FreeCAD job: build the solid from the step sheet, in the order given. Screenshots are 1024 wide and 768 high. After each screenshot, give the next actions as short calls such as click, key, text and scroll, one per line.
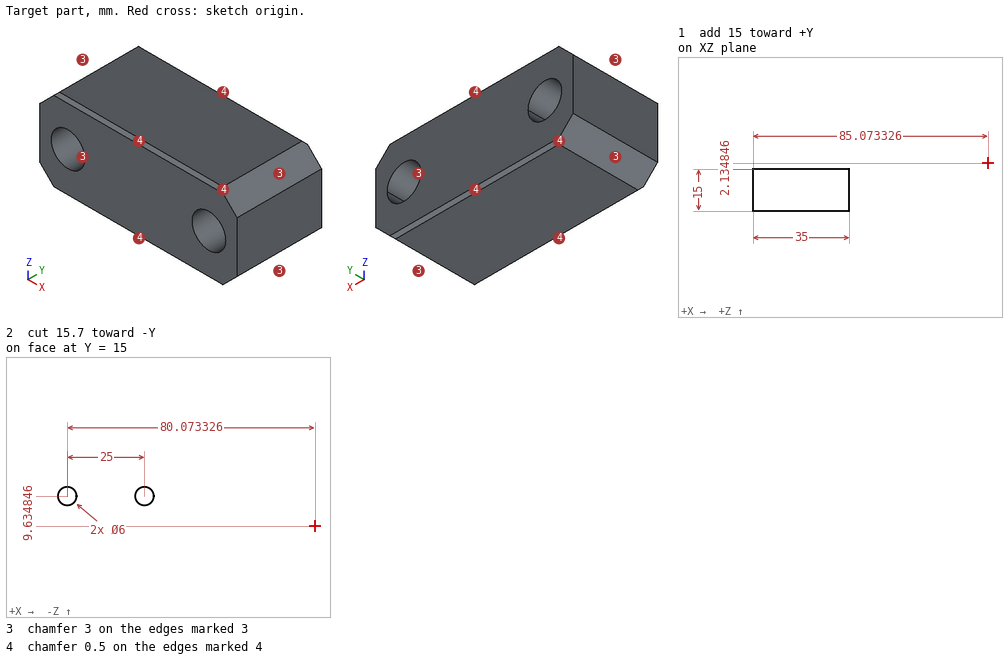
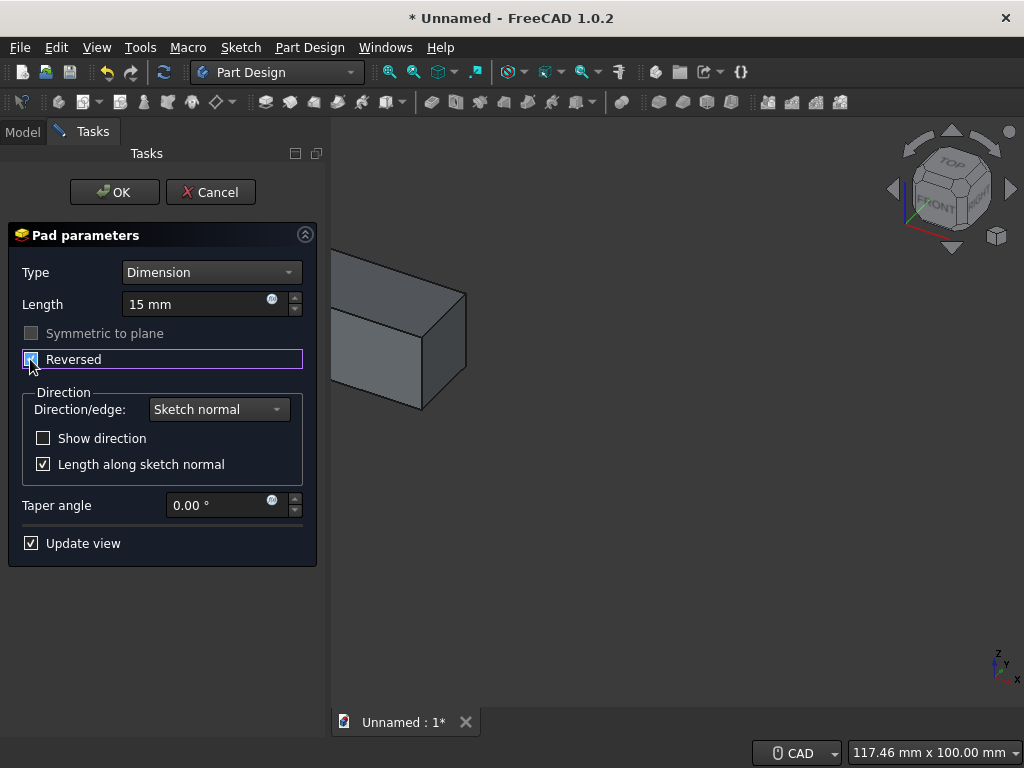
click(115, 192)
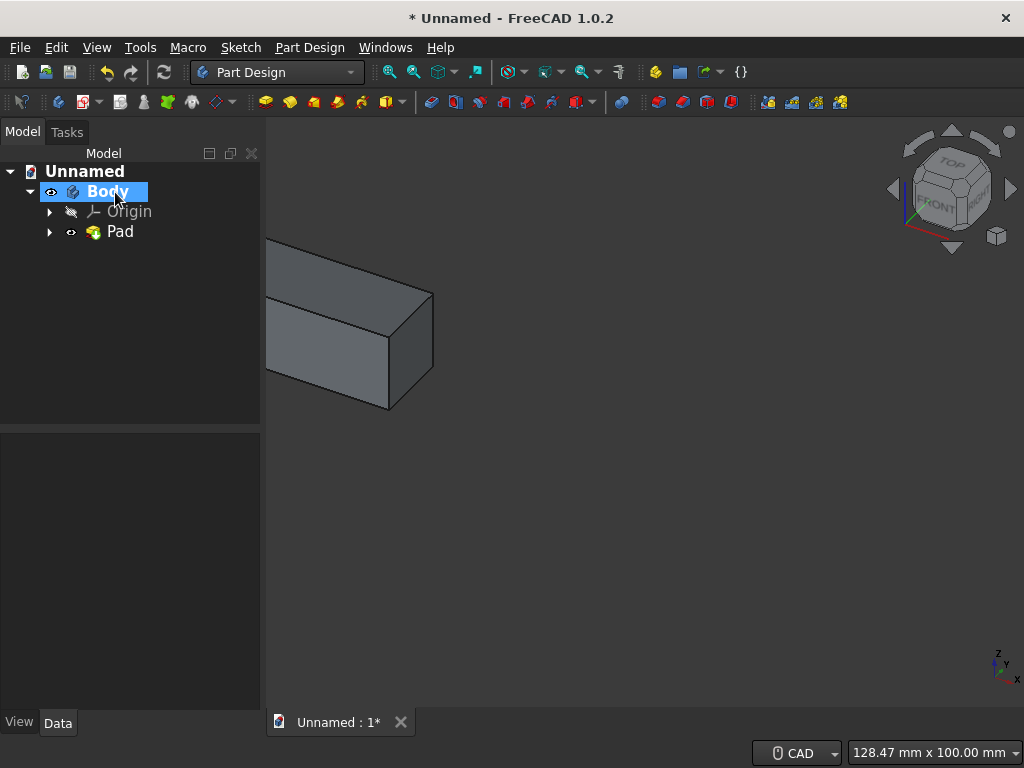
key(v)
key(f)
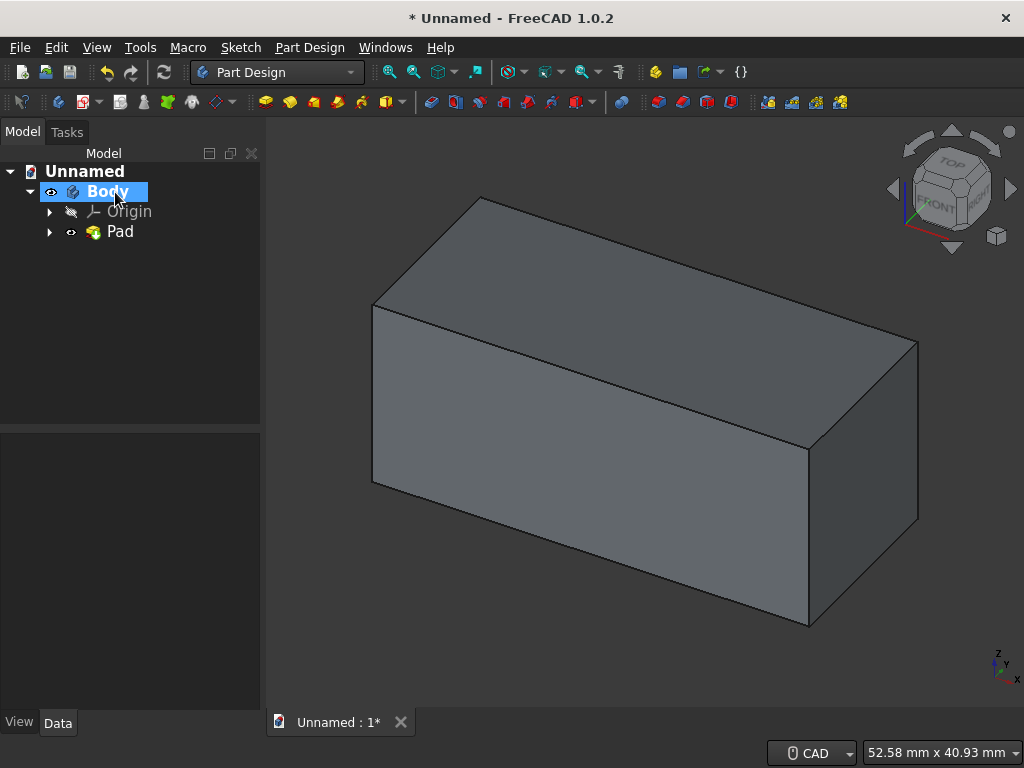
key(4)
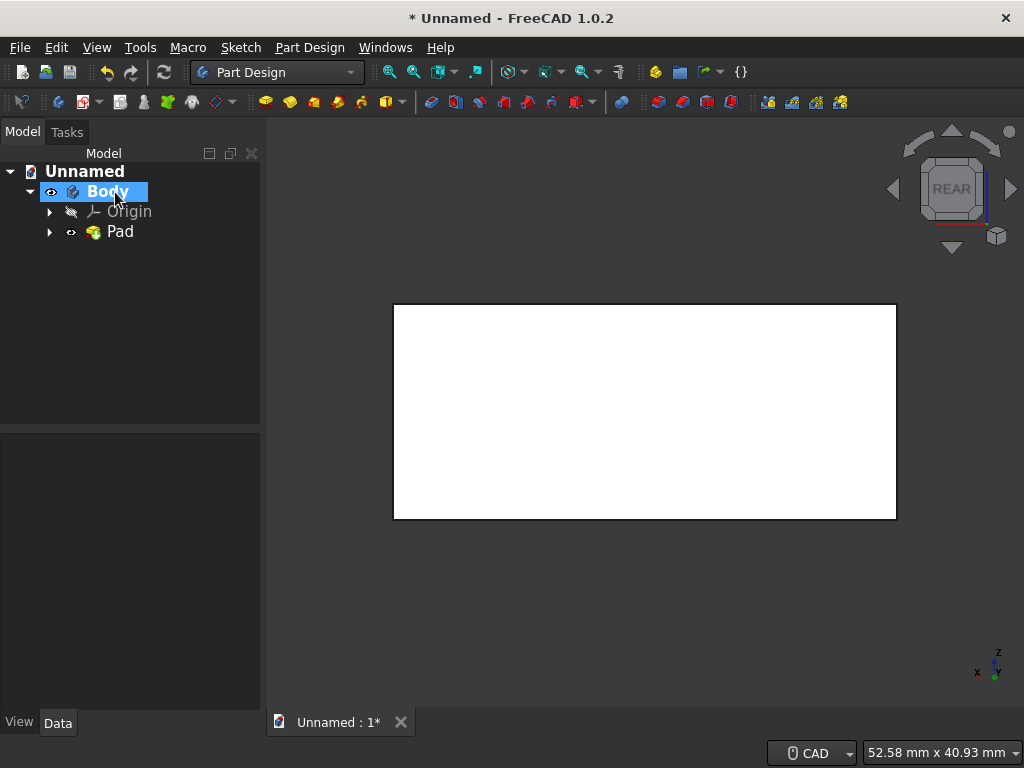
click(573, 411)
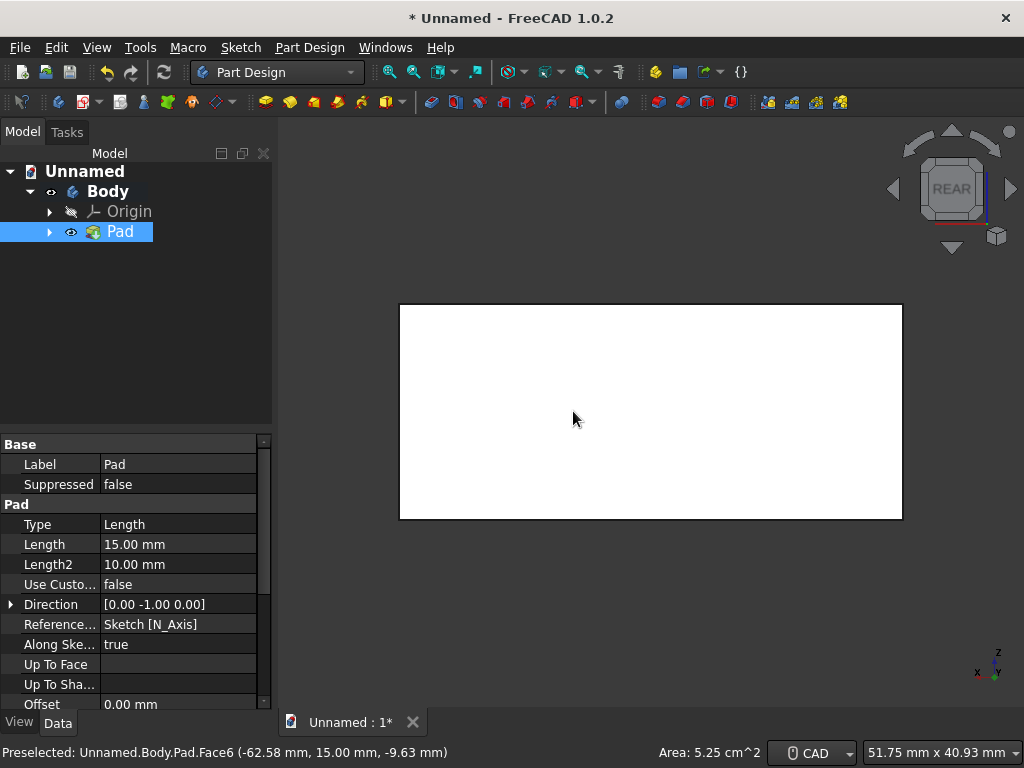
click(84, 102)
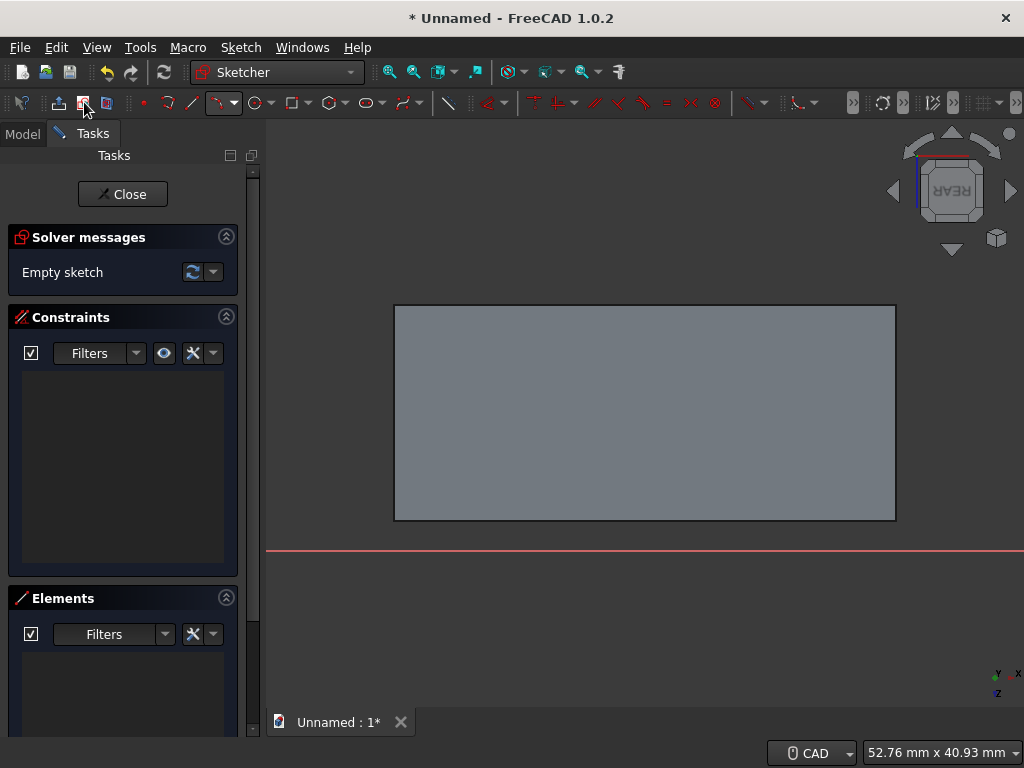
scroll(294, 413, down, 1)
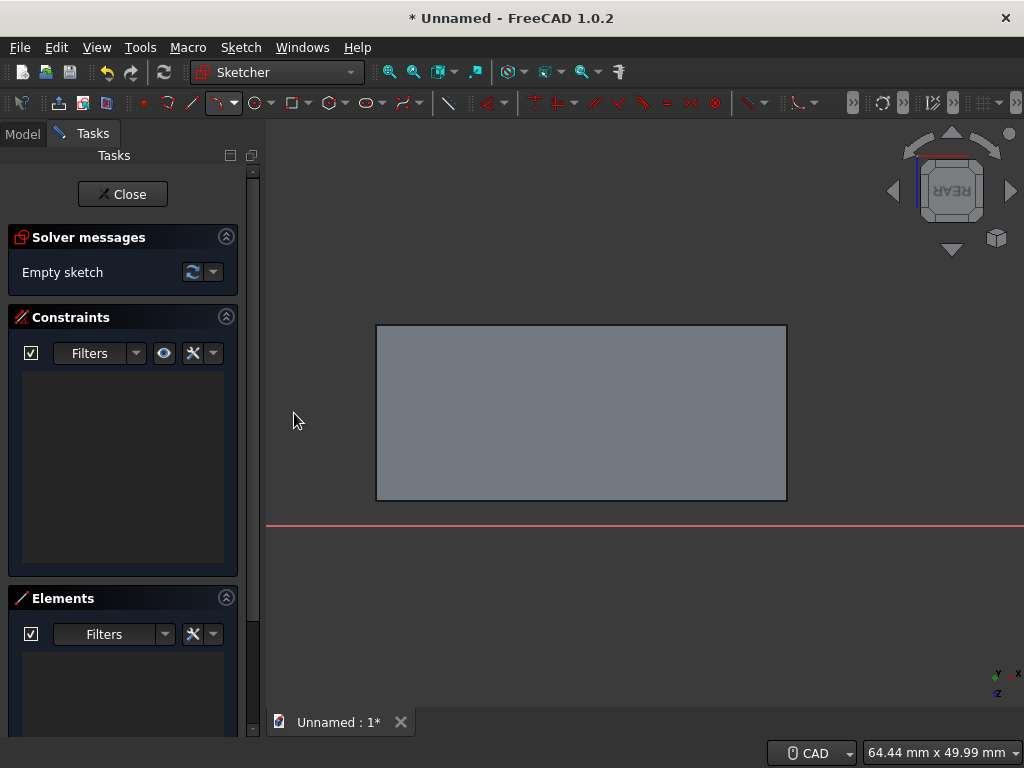
key(g)
key(c)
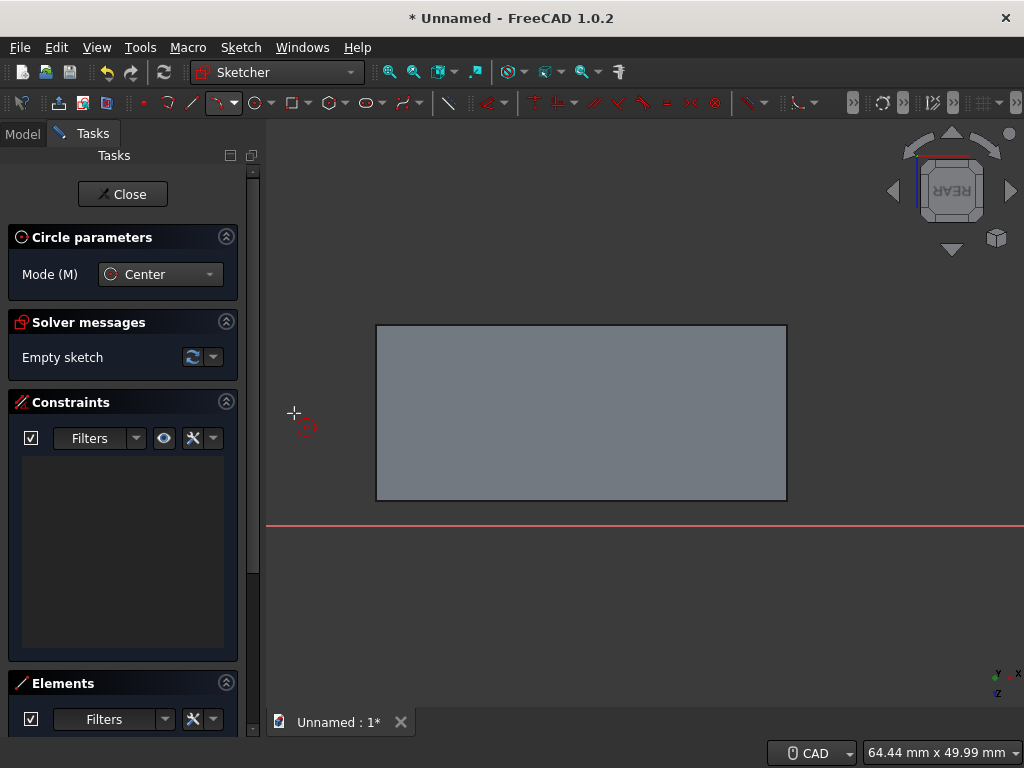
click(434, 413)
click(459, 388)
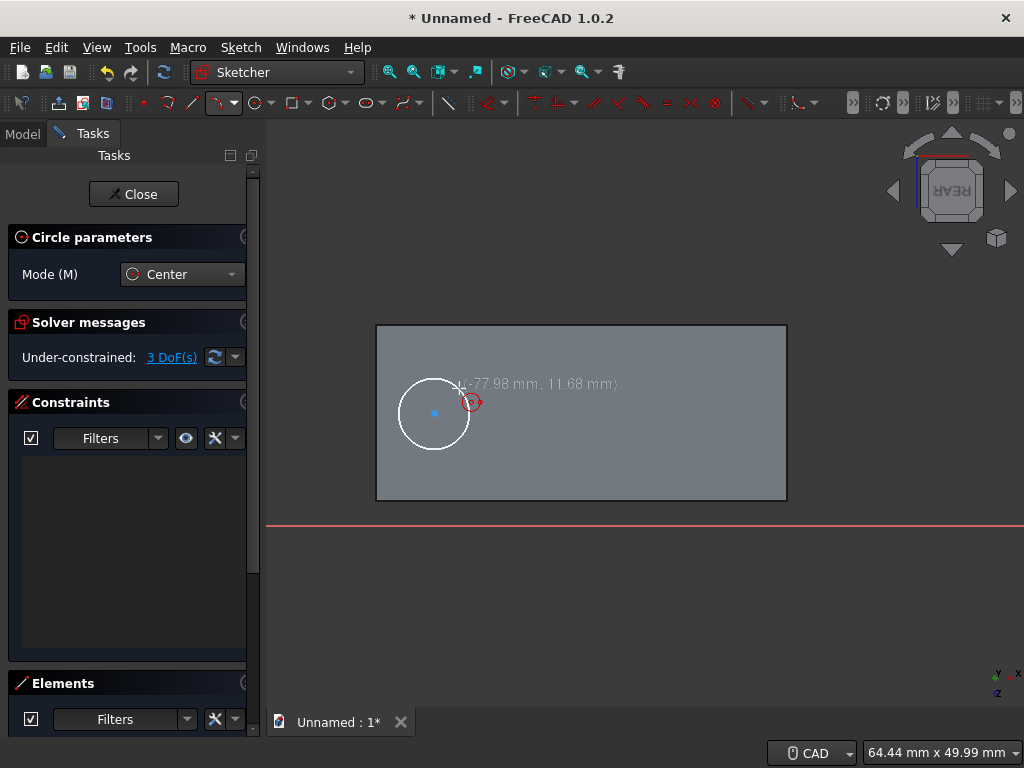
click(728, 413)
click(753, 388)
key(Escape)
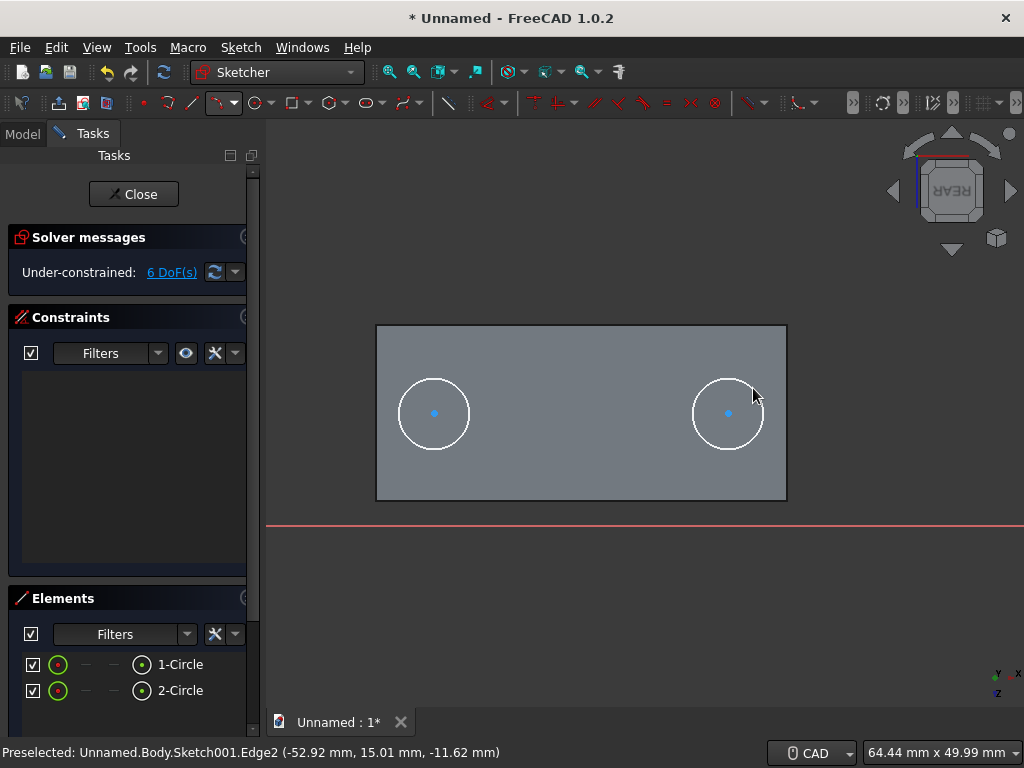
click(459, 389)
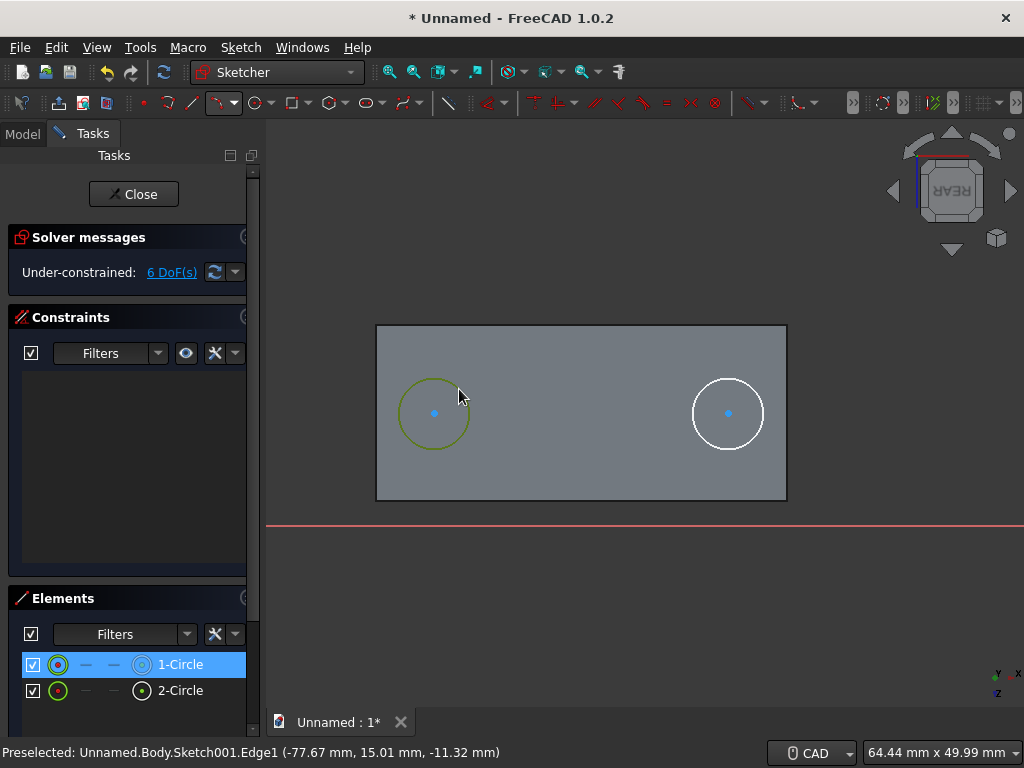
click(753, 389)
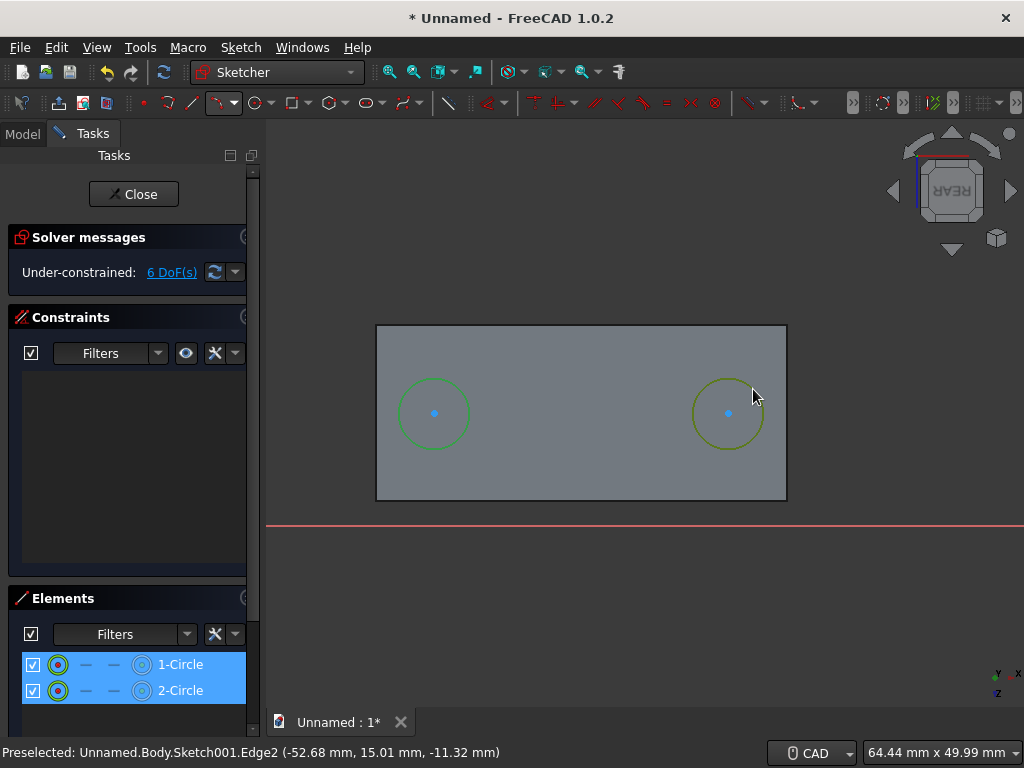
key(e)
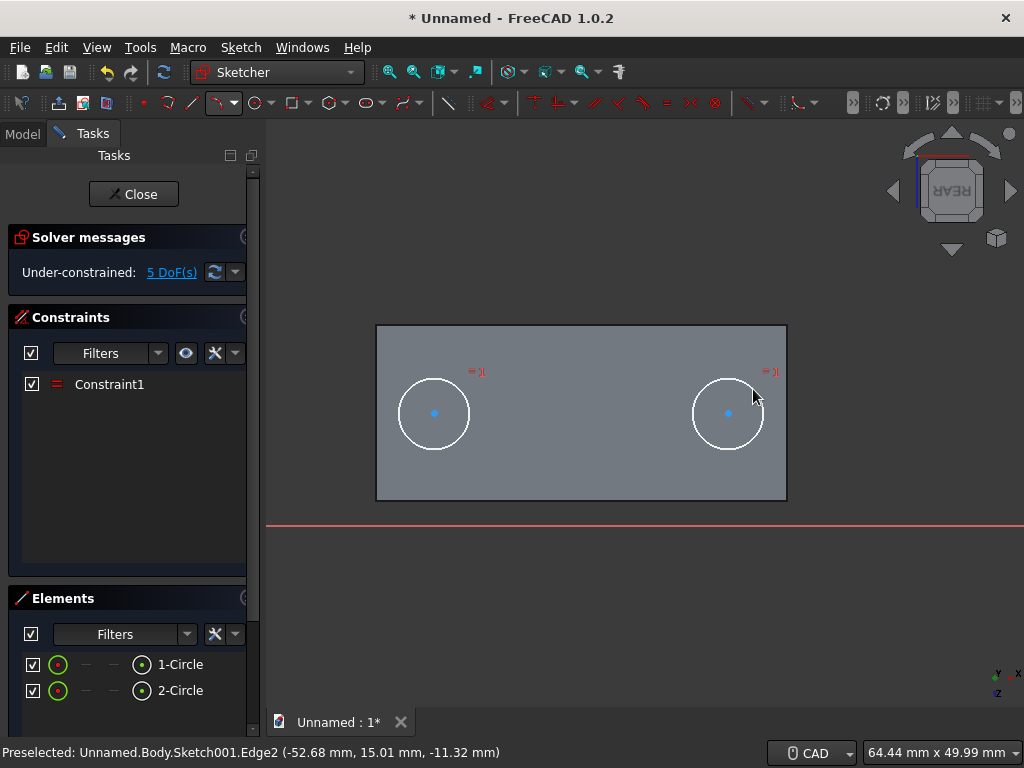
click(434, 414)